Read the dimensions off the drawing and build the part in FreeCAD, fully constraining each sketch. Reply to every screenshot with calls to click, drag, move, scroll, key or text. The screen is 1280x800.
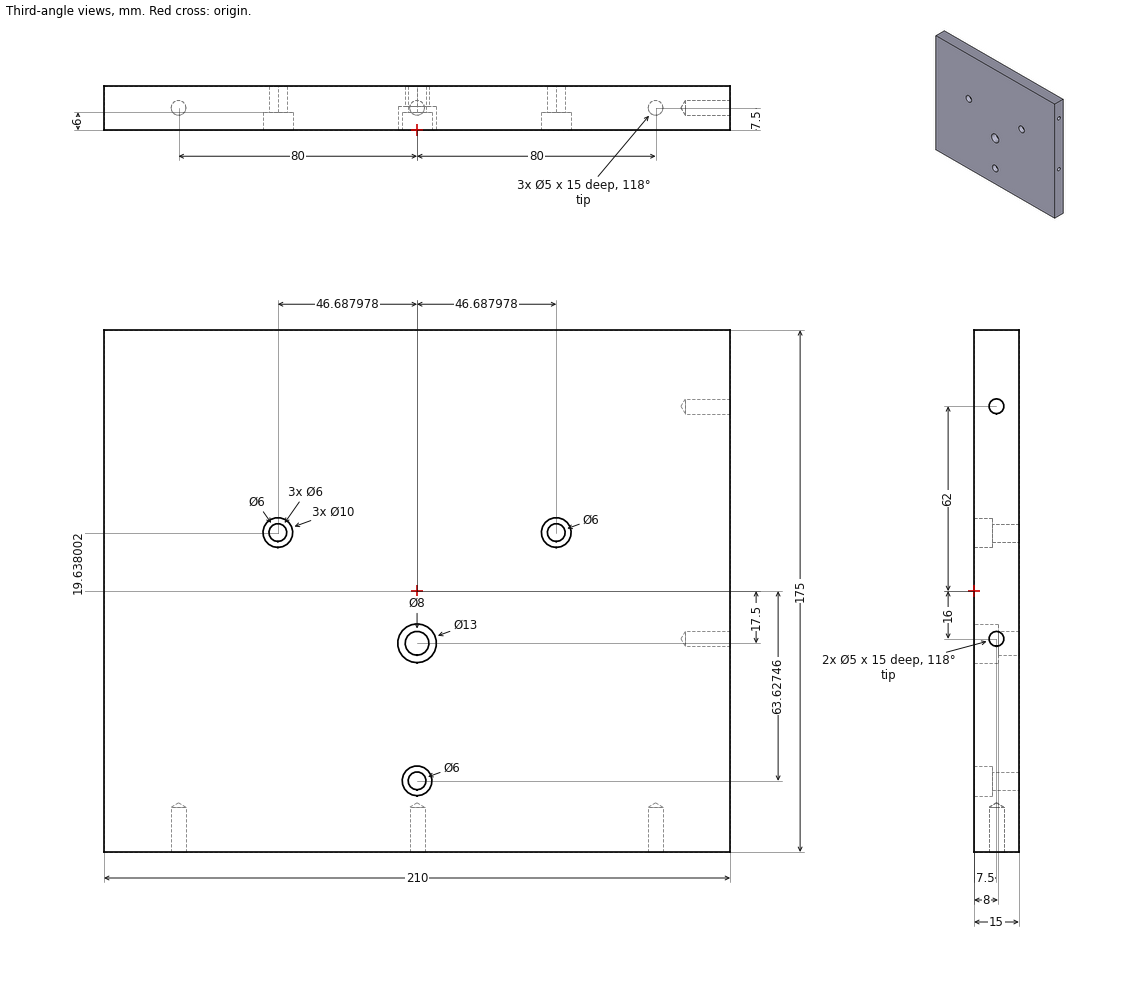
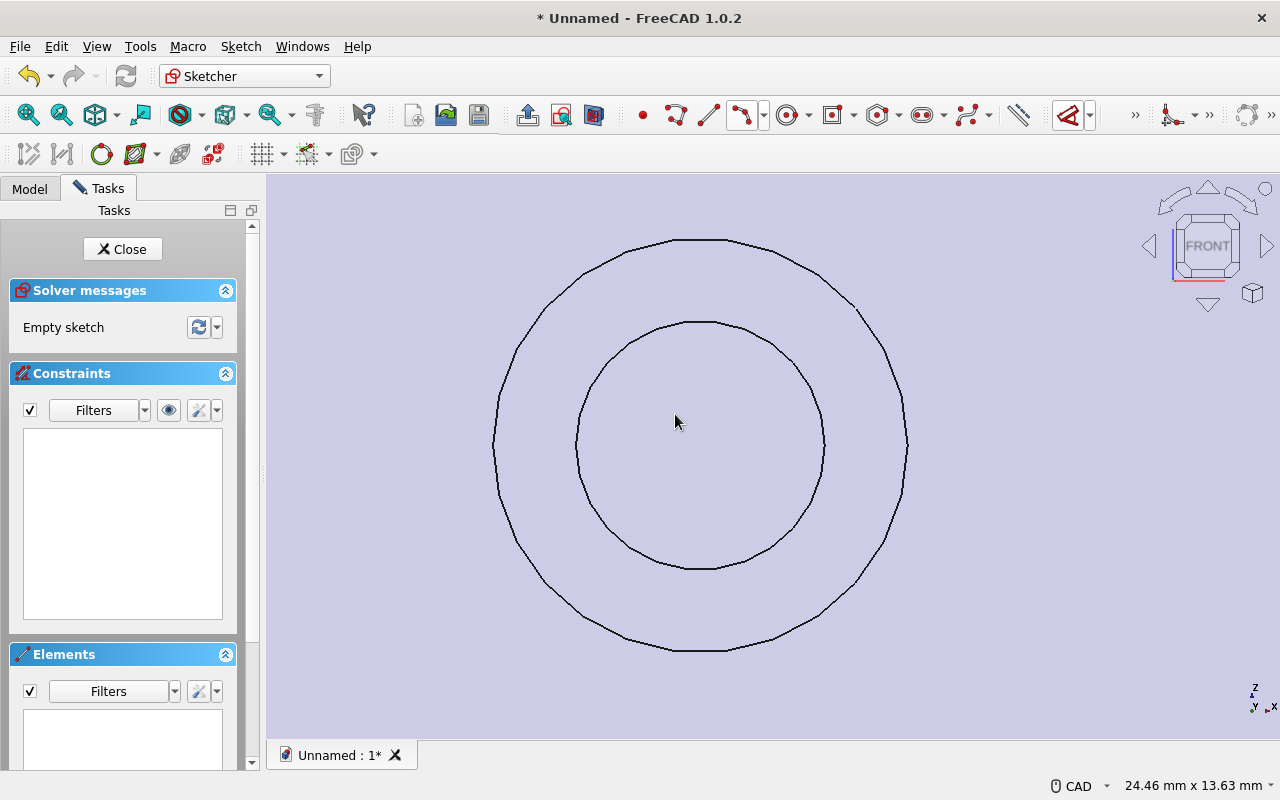
scroll(692, 423, up, 2)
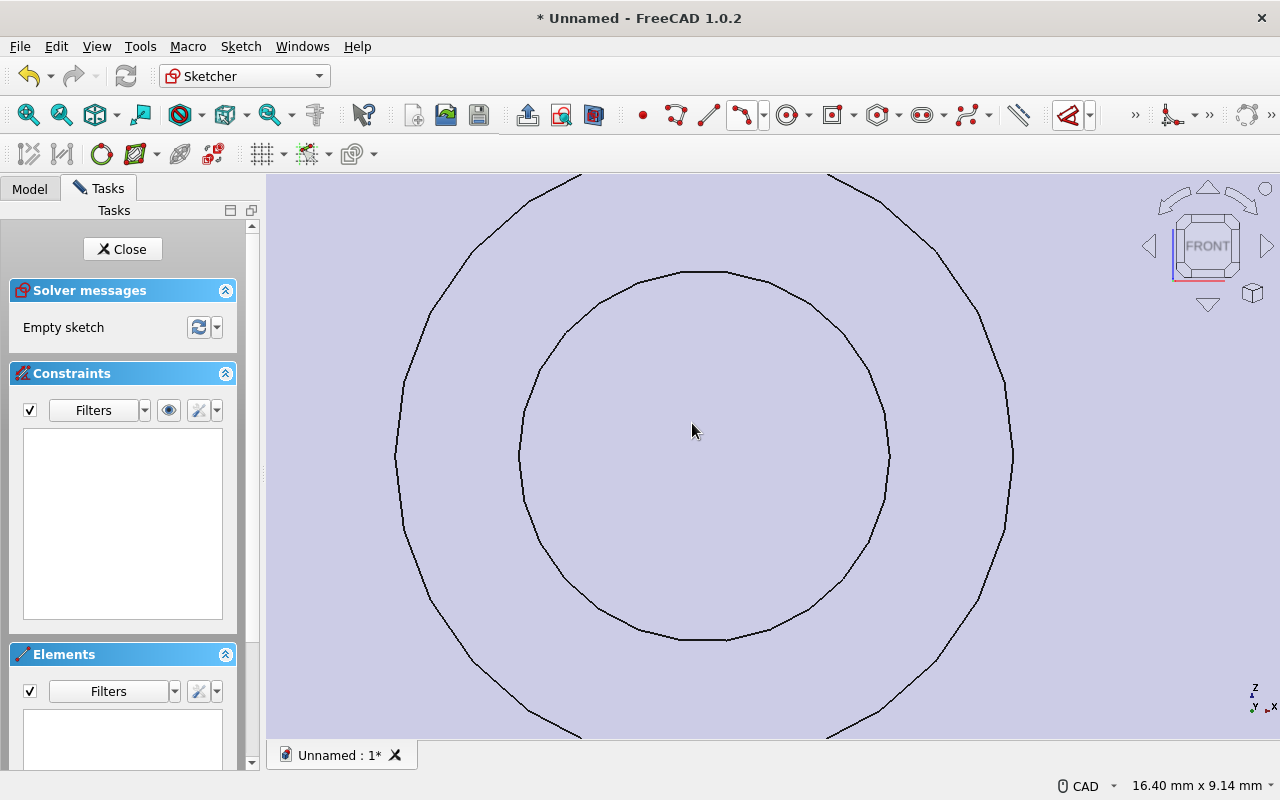
click(786, 116)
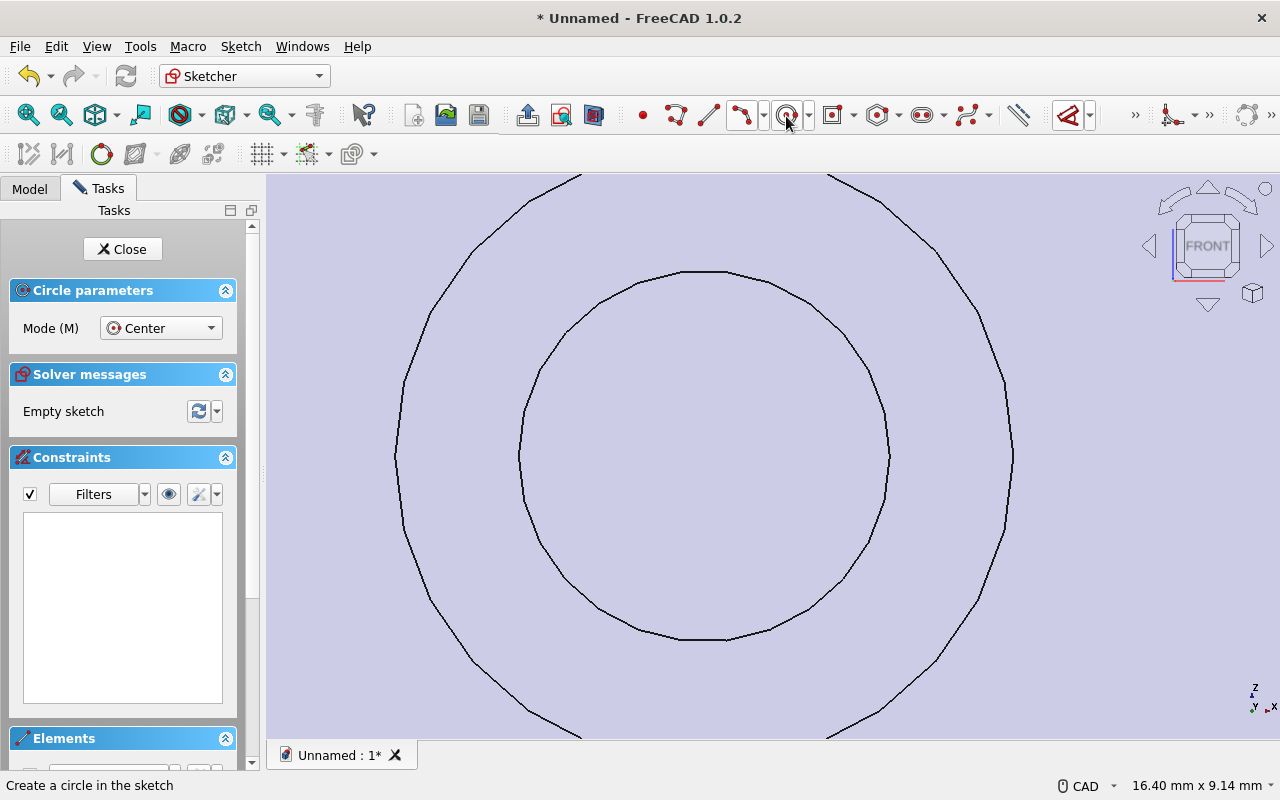
click(704, 456)
click(835, 325)
key(Escape)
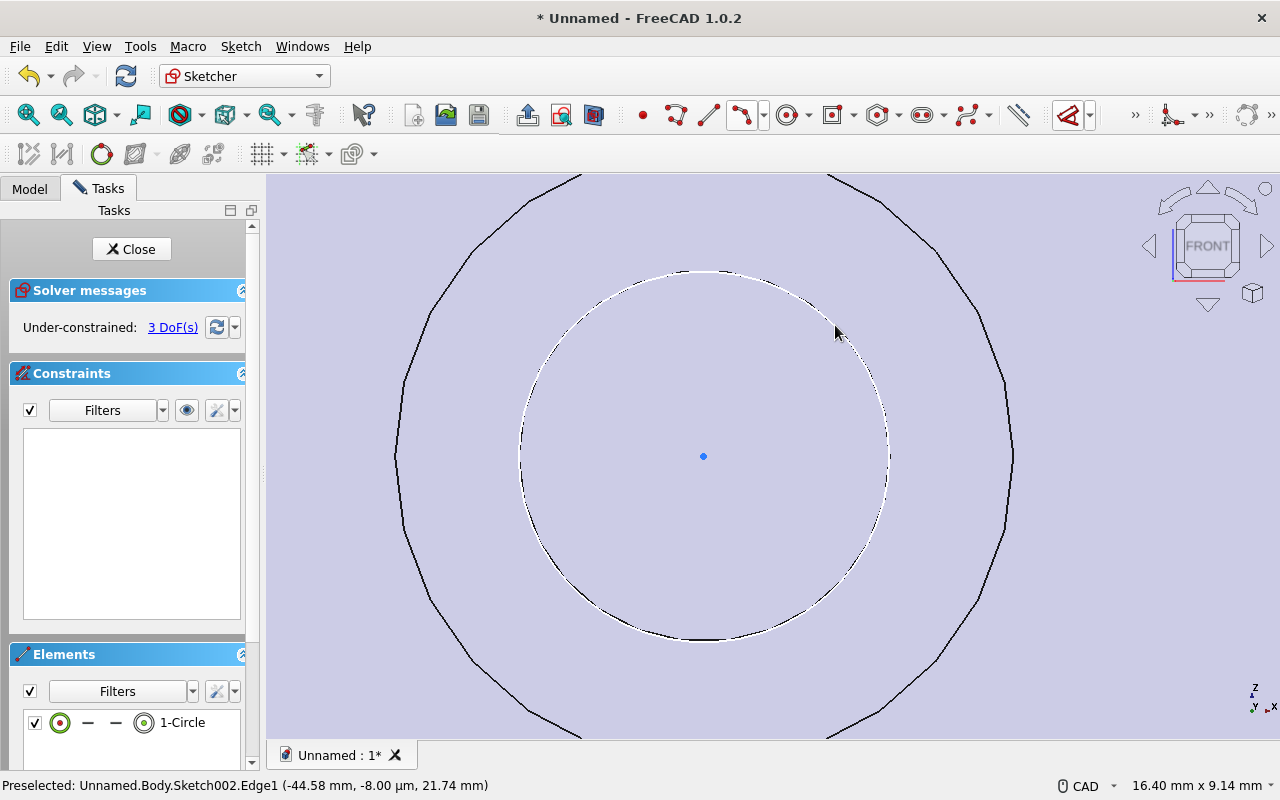
click(835, 326)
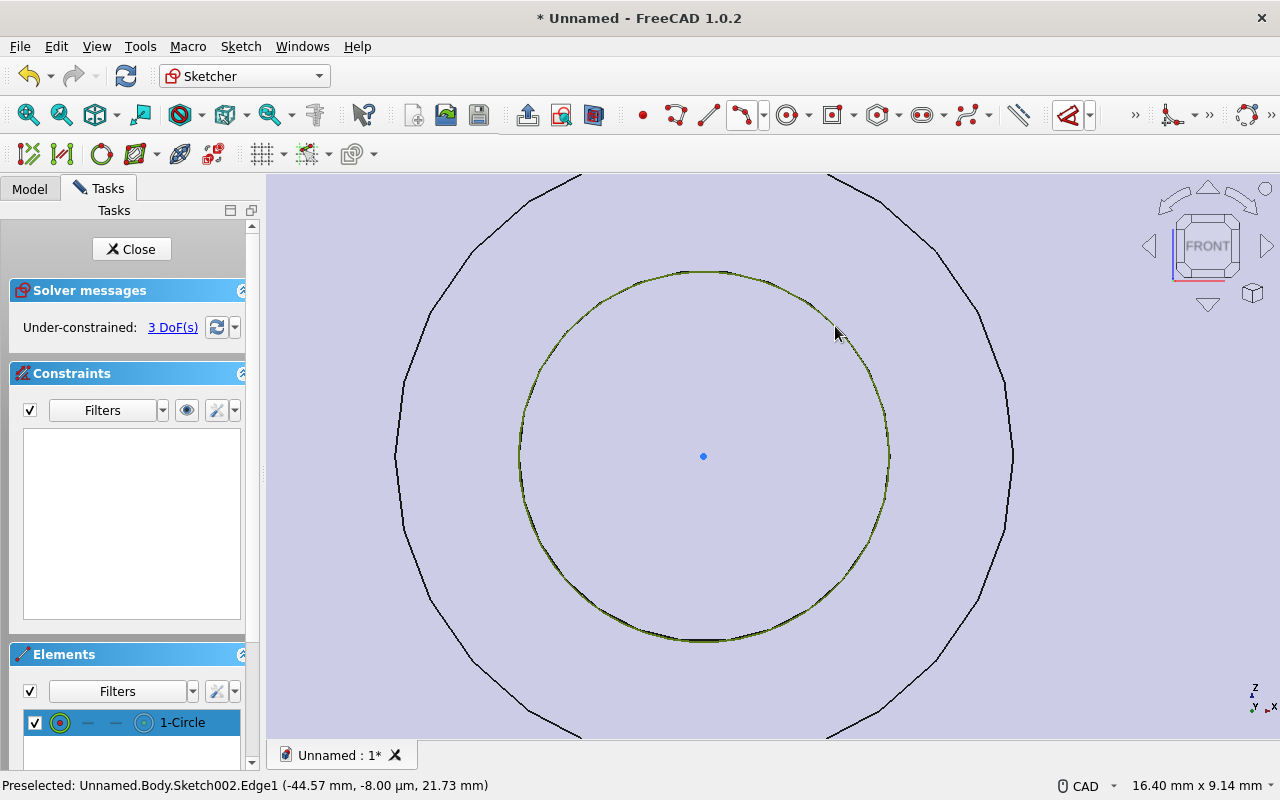
key(k)
key(o)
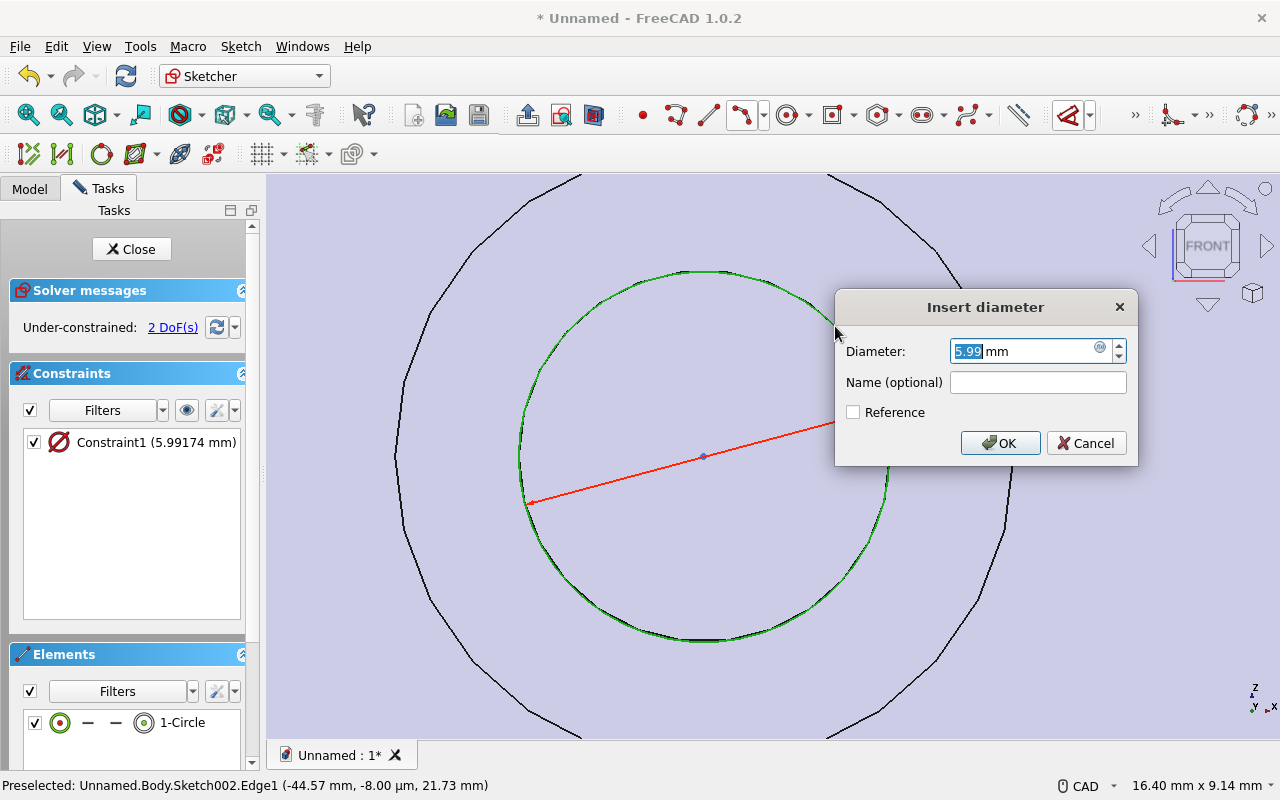
text(6)
key(Return)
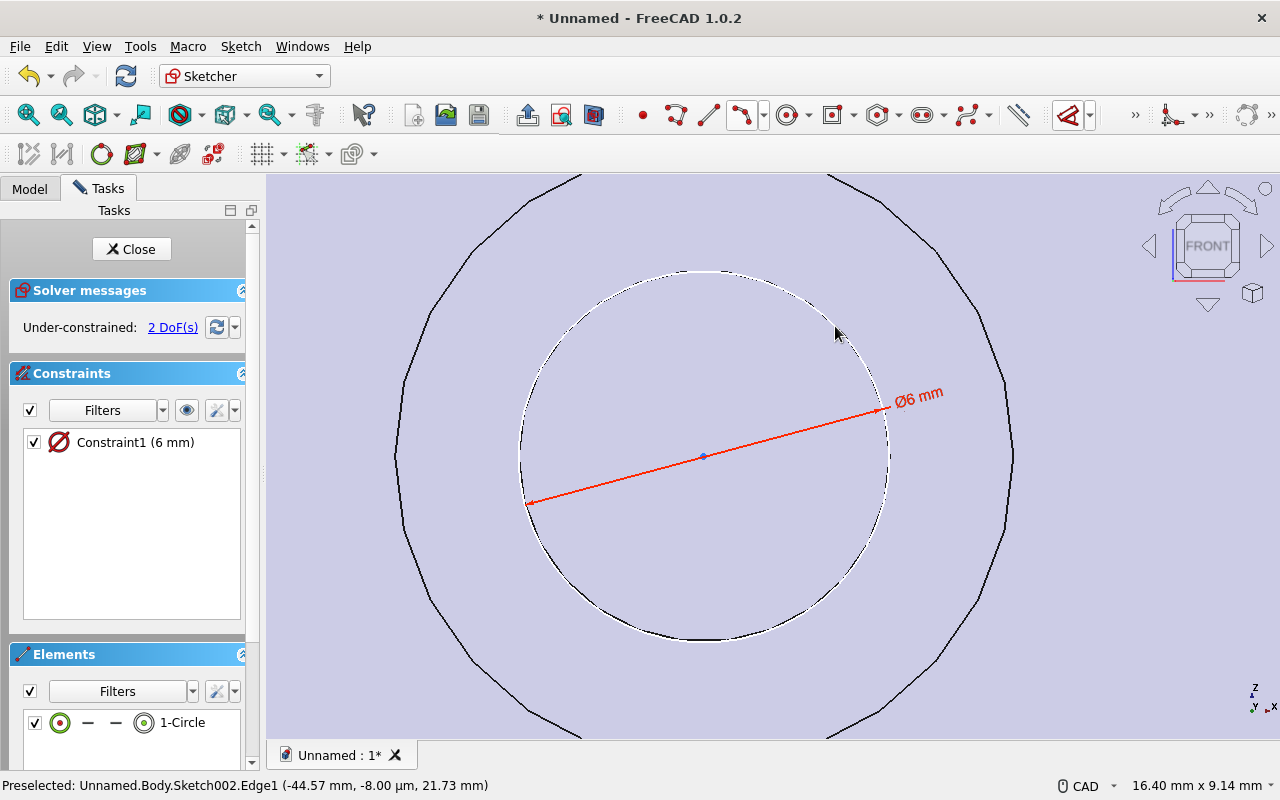
click(704, 457)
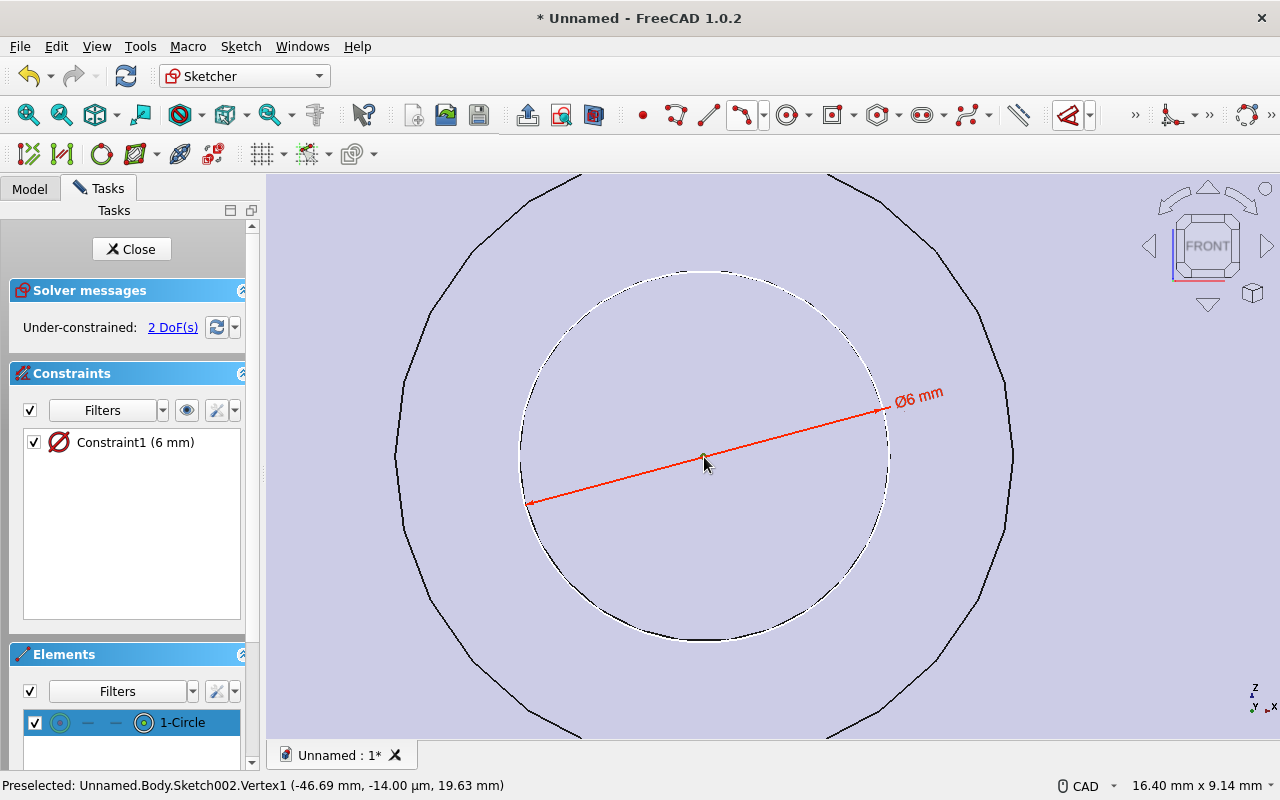
key(l)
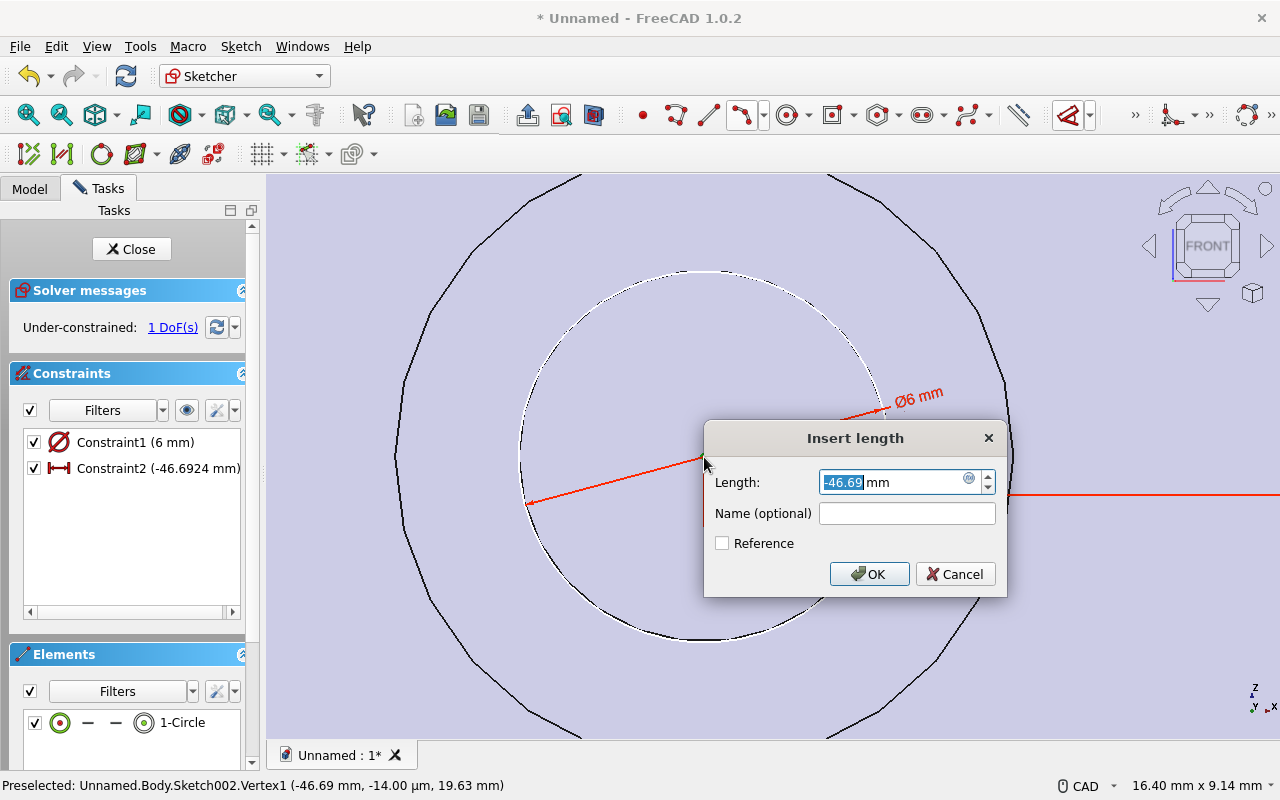
text(-46.687978)
key(Return)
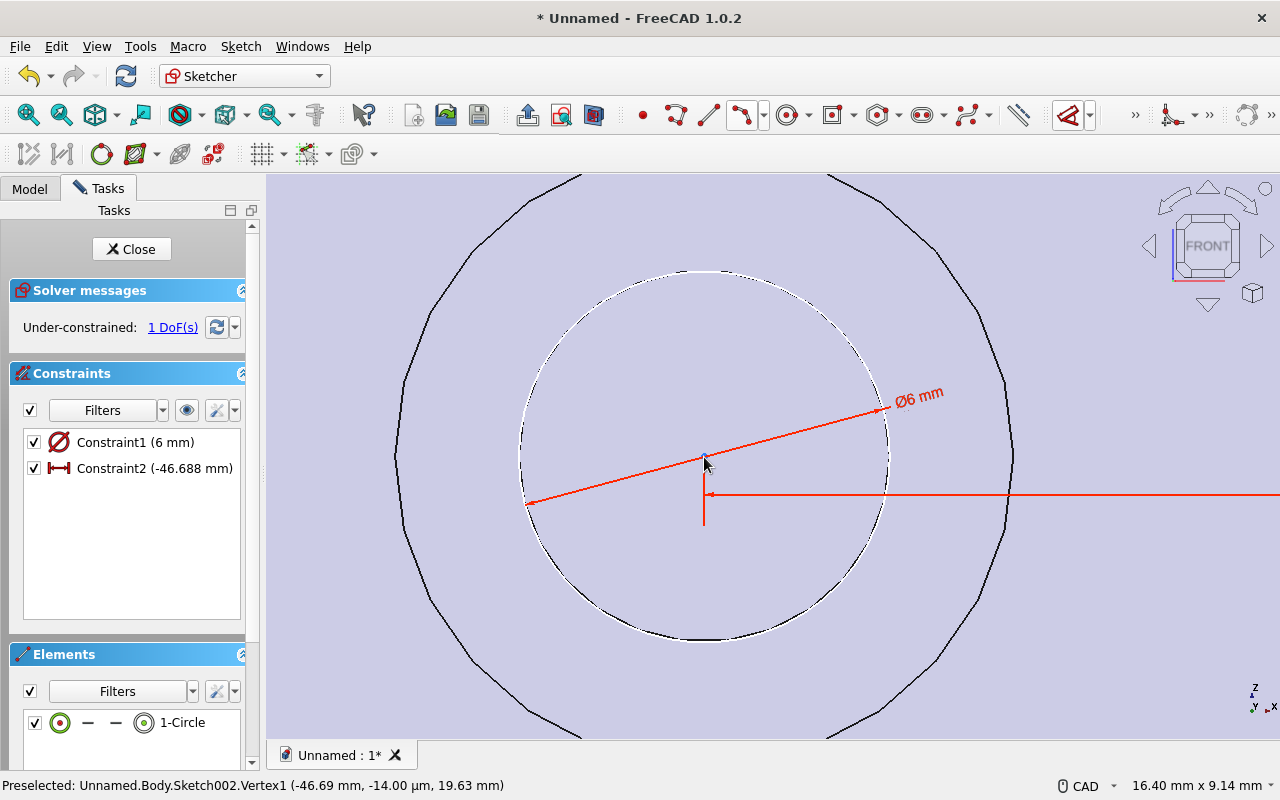
click(704, 457)